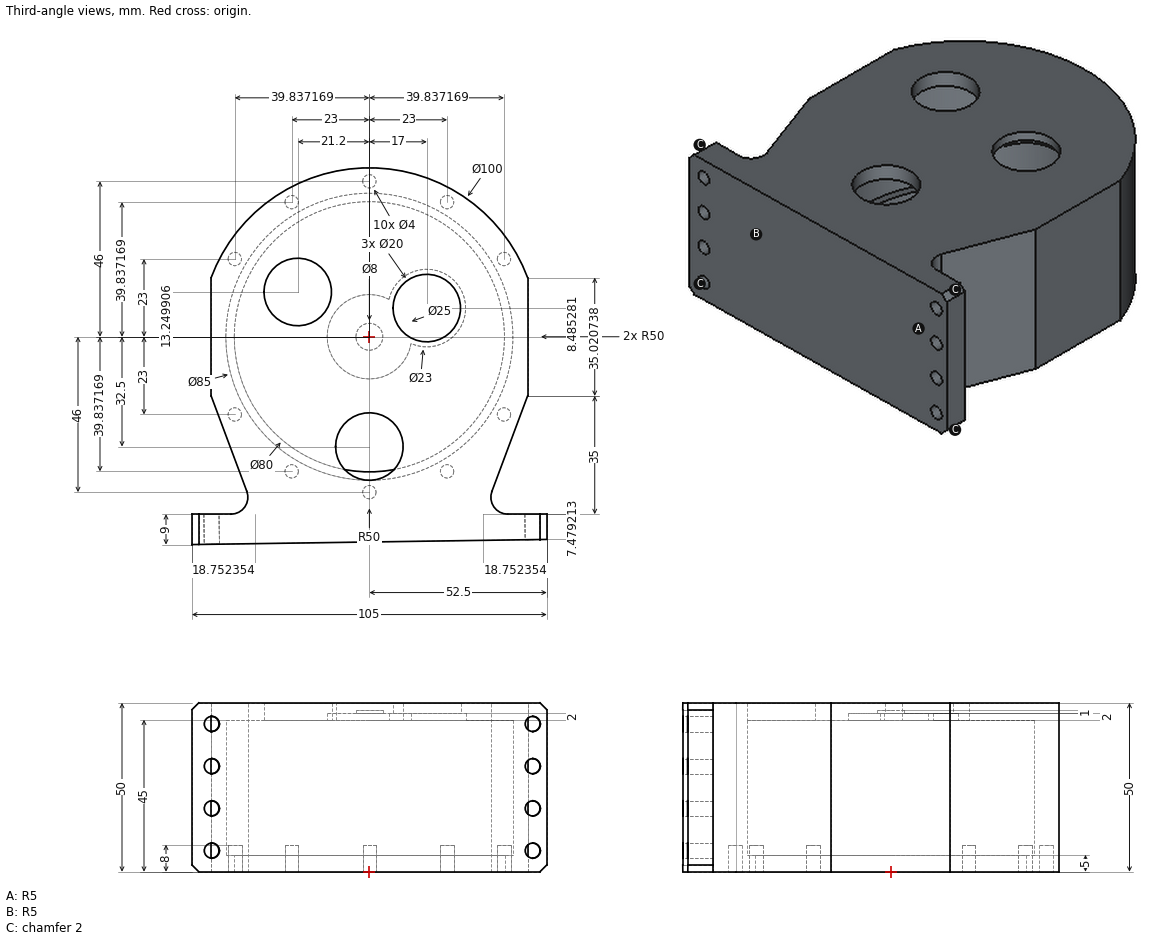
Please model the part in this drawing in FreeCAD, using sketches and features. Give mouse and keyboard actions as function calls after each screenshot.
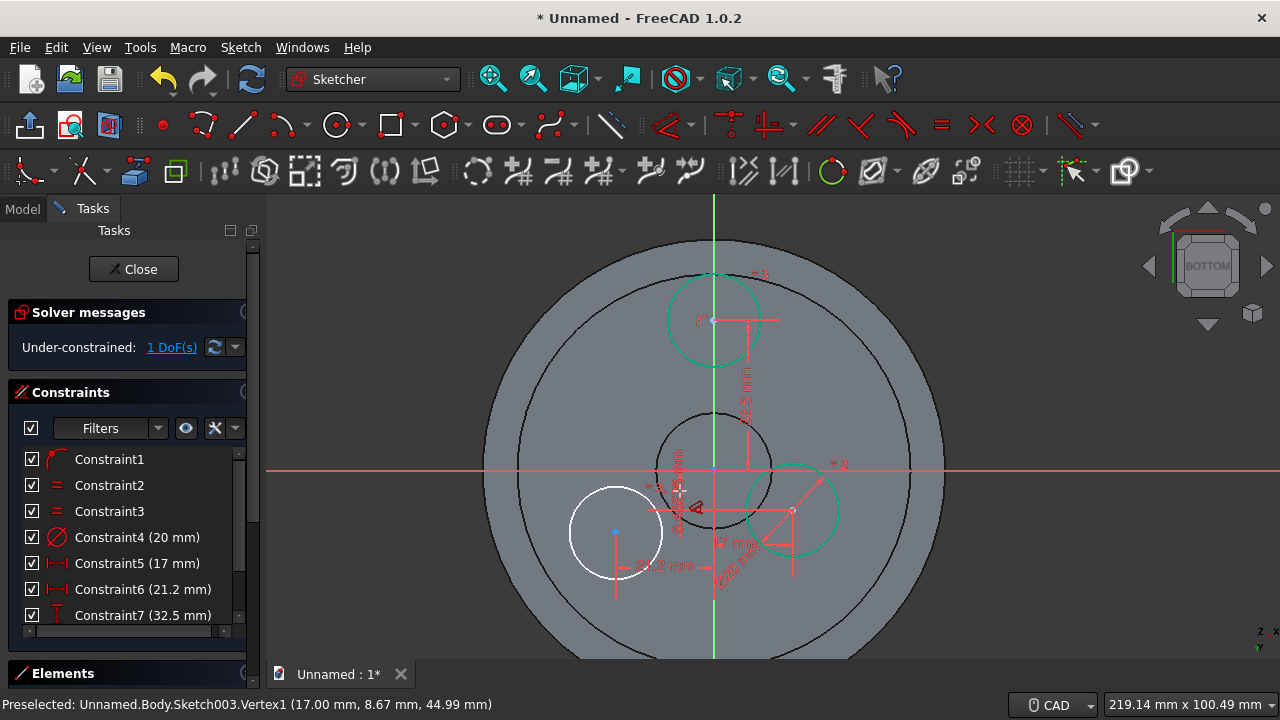
click(616, 533)
click(558, 502)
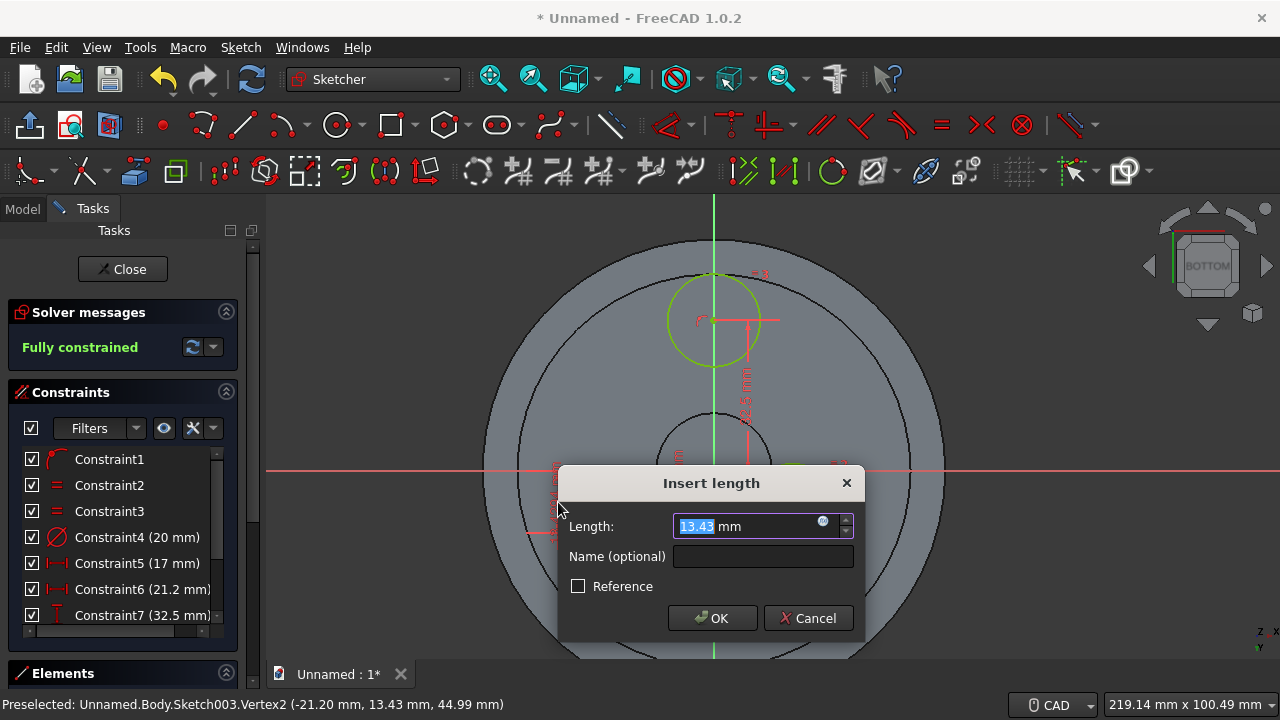
text(13.249906)
key(Return)
key(Escape)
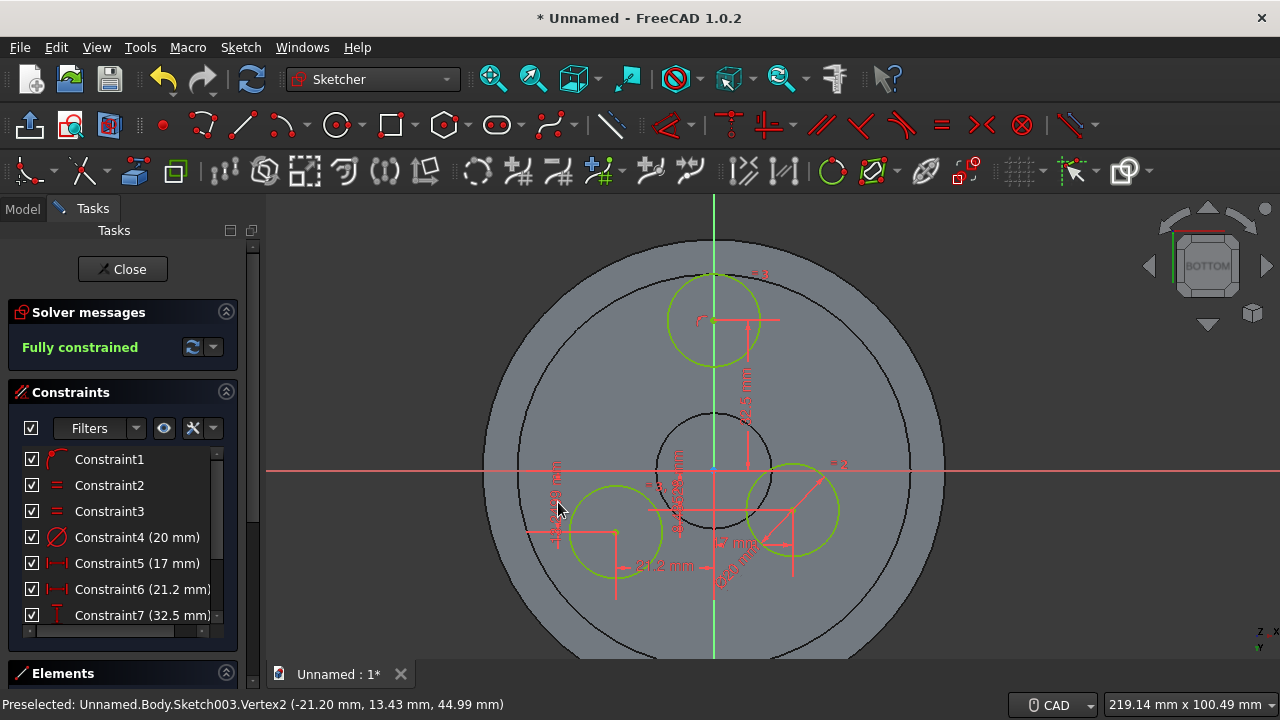
click(123, 269)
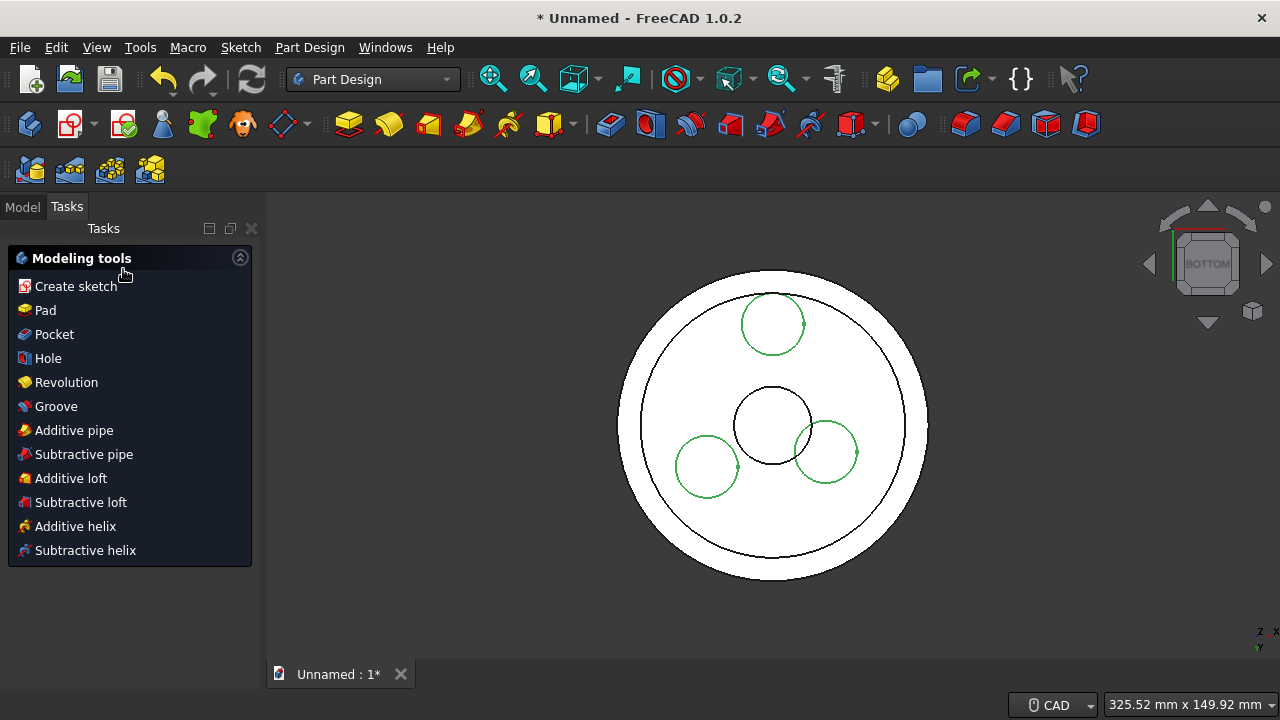
click(612, 124)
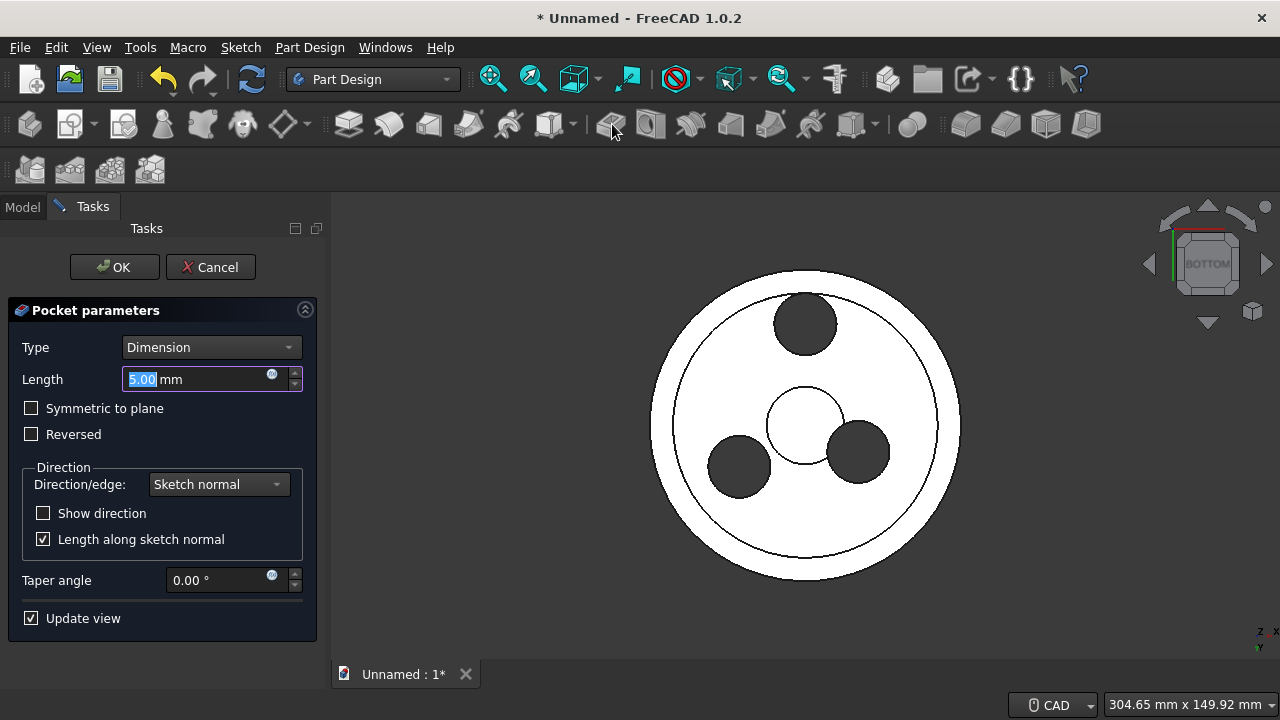
click(212, 348)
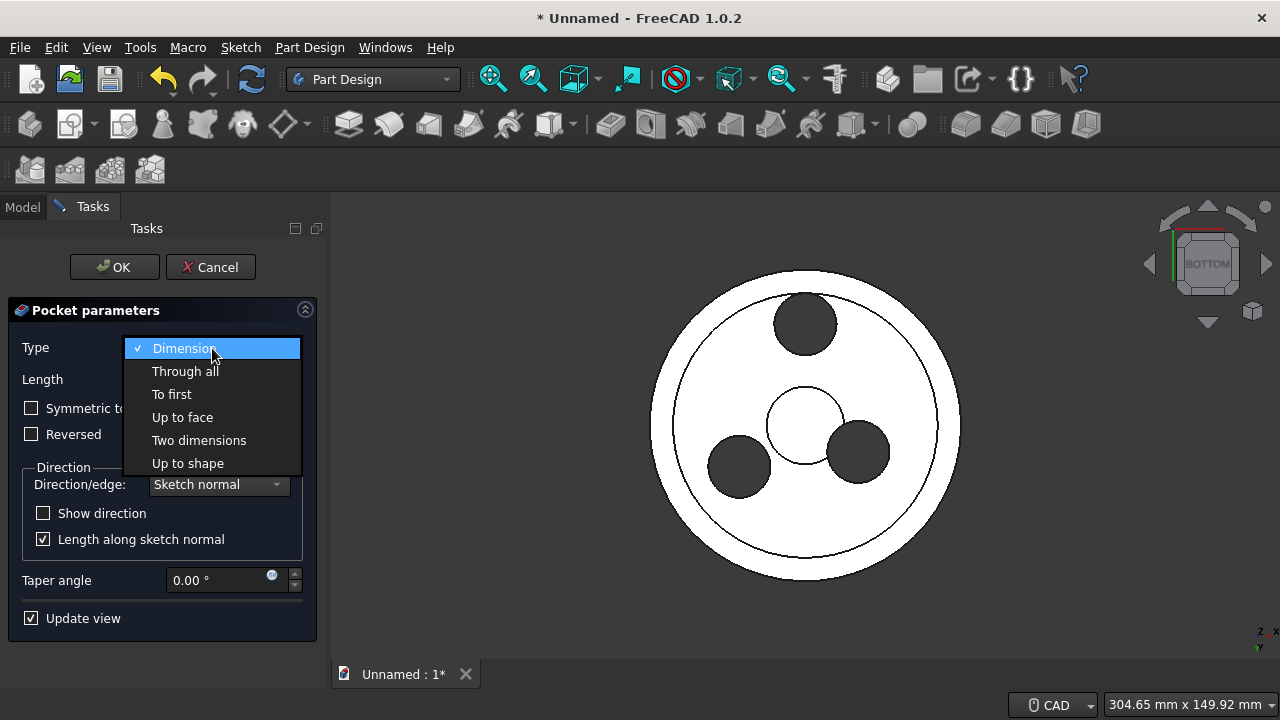
click(212, 372)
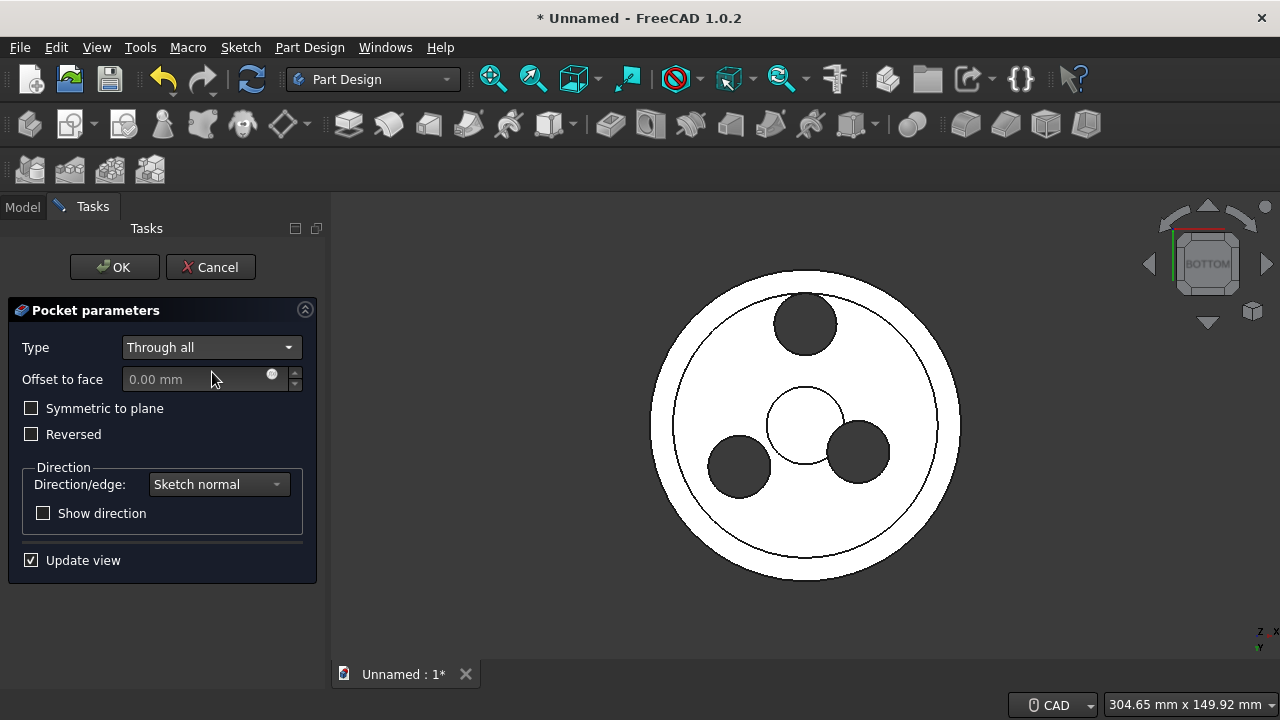
click(115, 267)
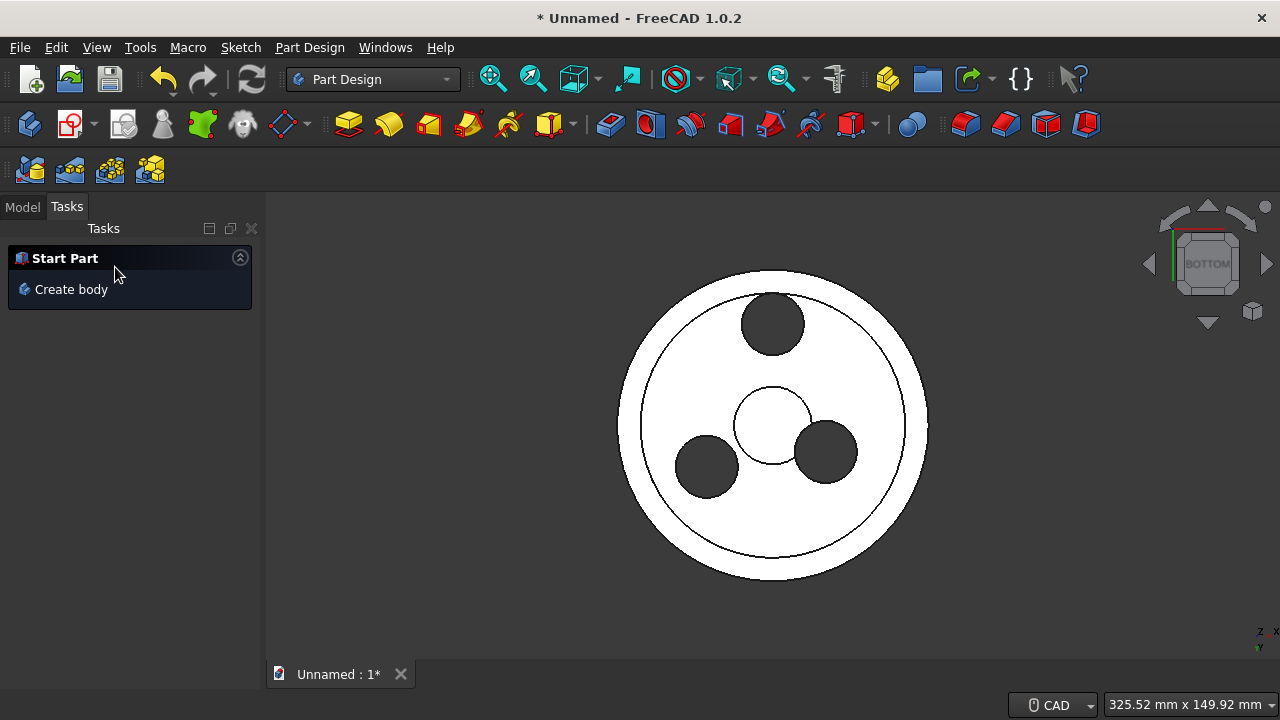
click(70, 124)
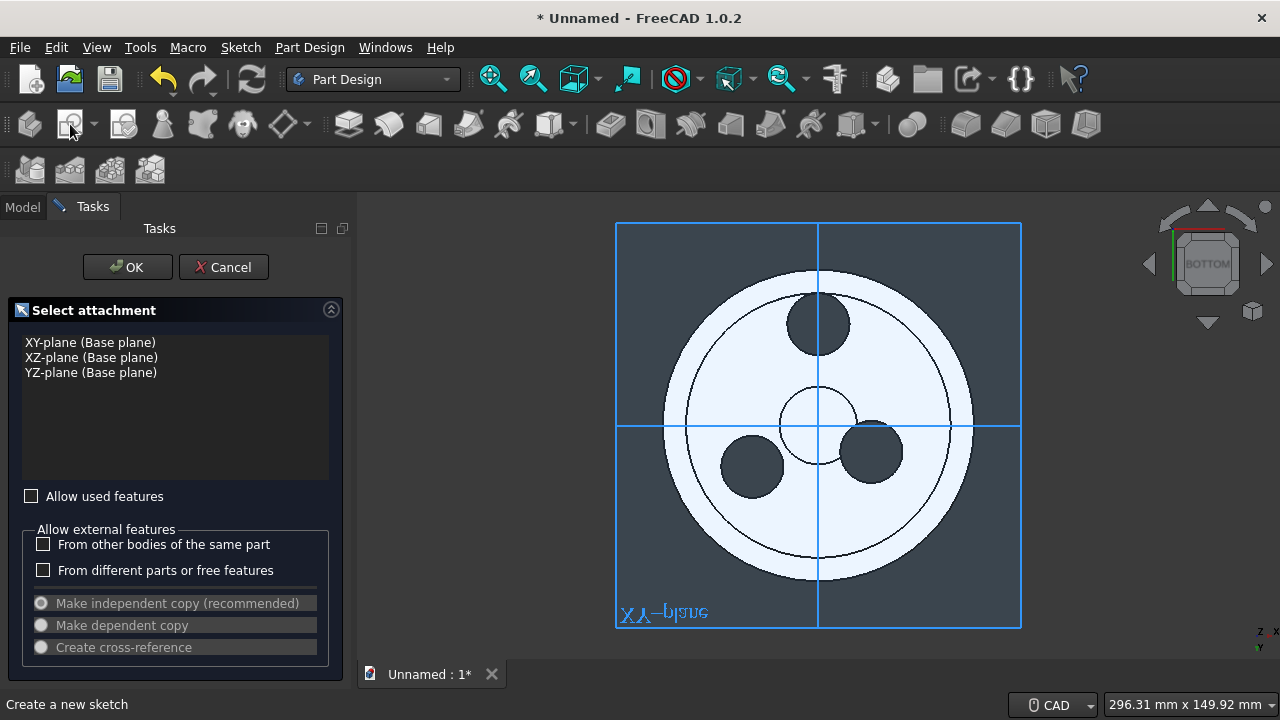
click(82, 342)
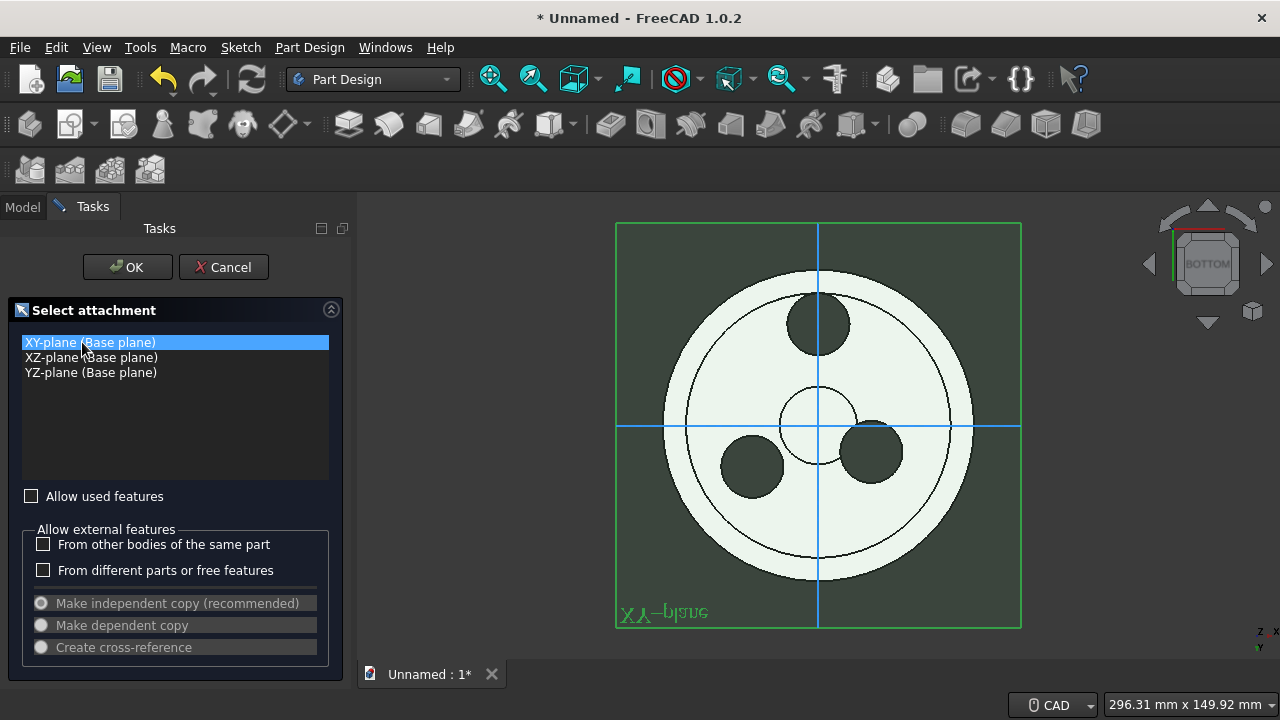
click(128, 267)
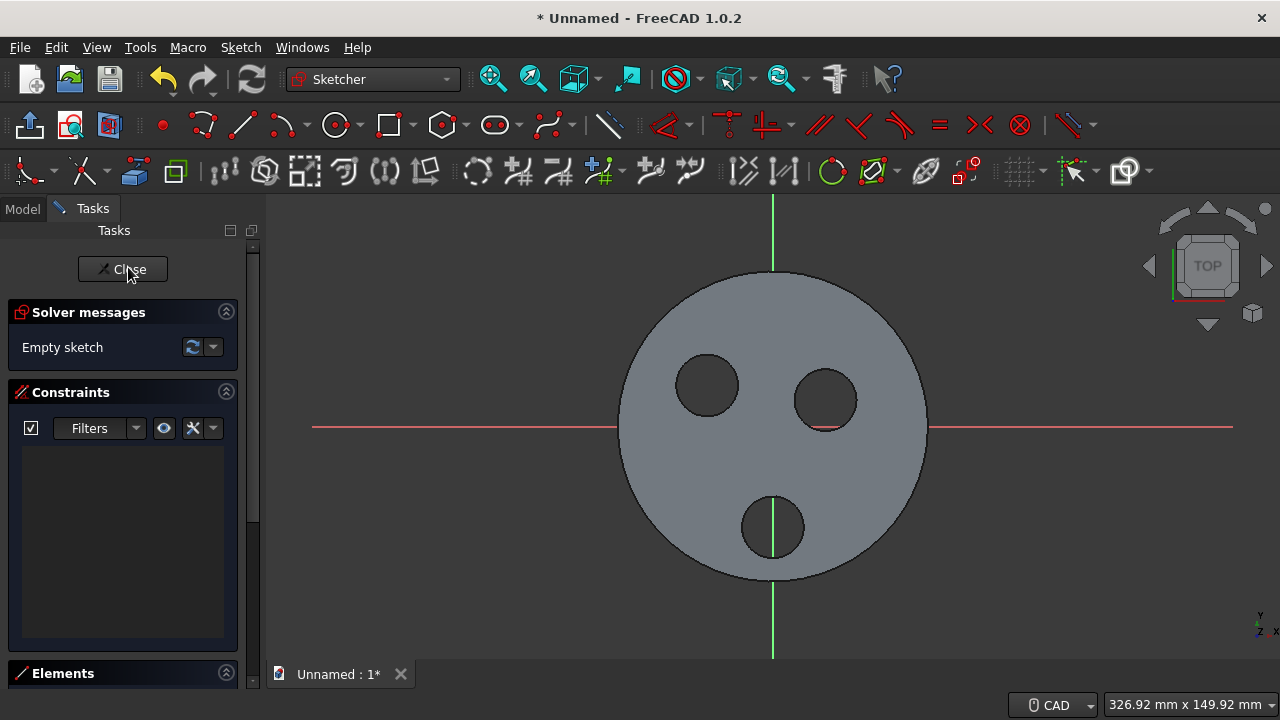
click(110, 126)